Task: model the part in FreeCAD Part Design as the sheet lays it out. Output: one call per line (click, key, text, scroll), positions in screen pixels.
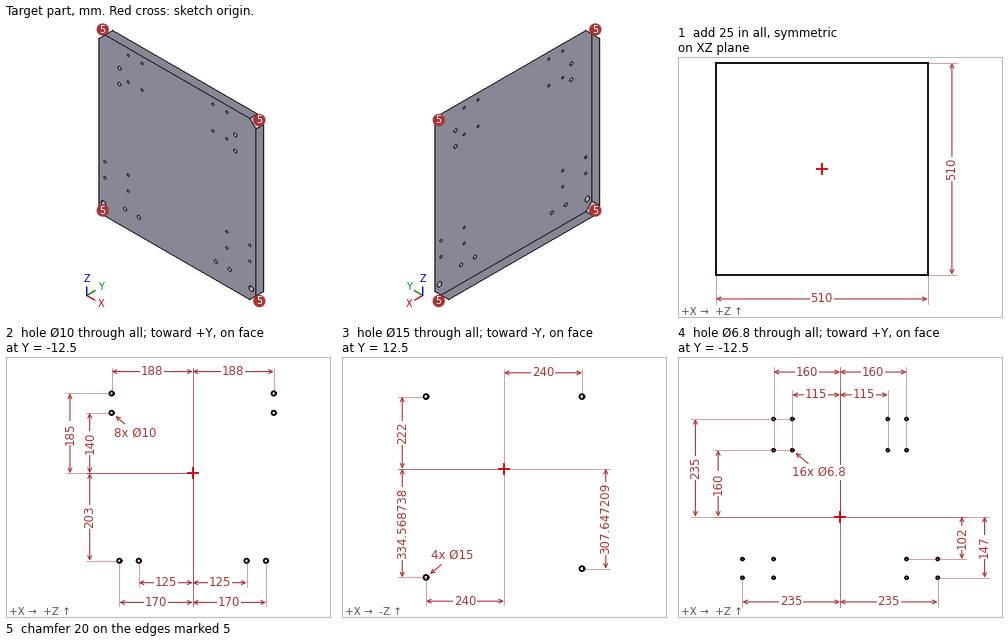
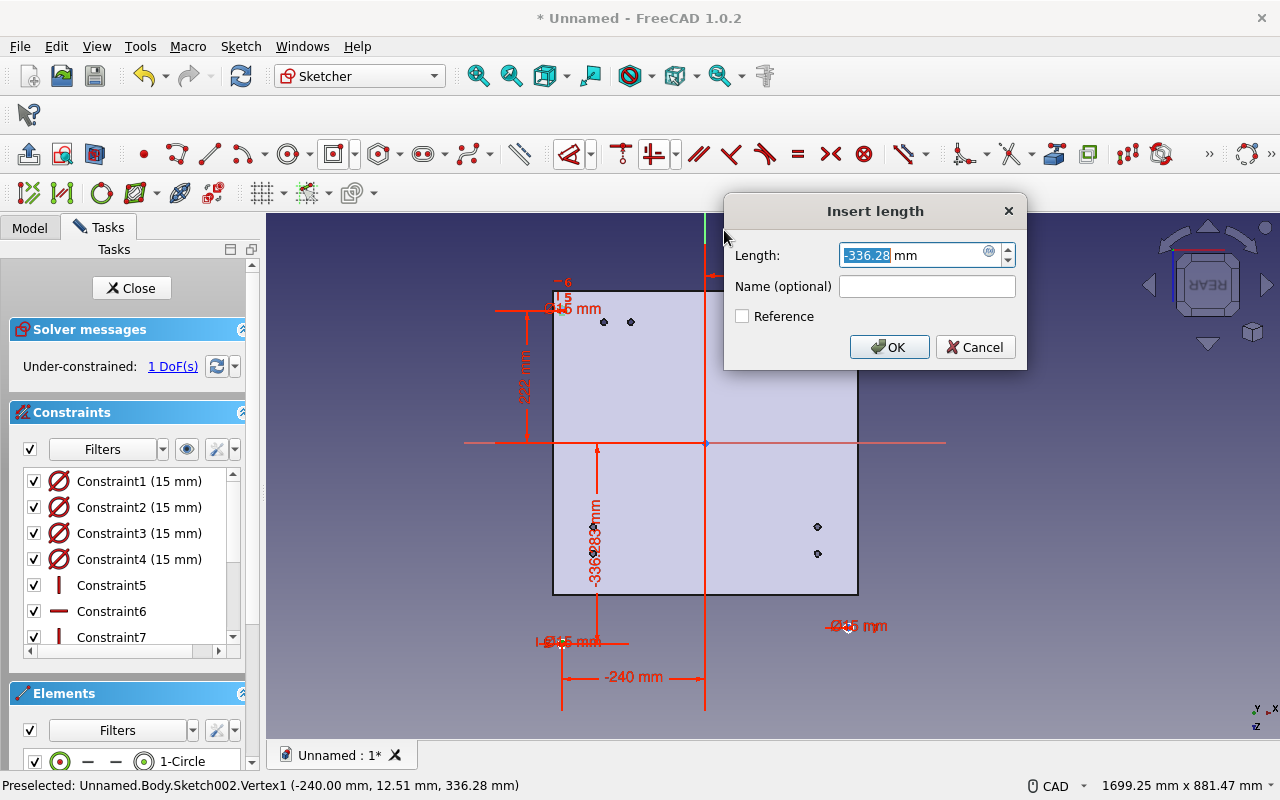
text(-334.568738)
key(Return)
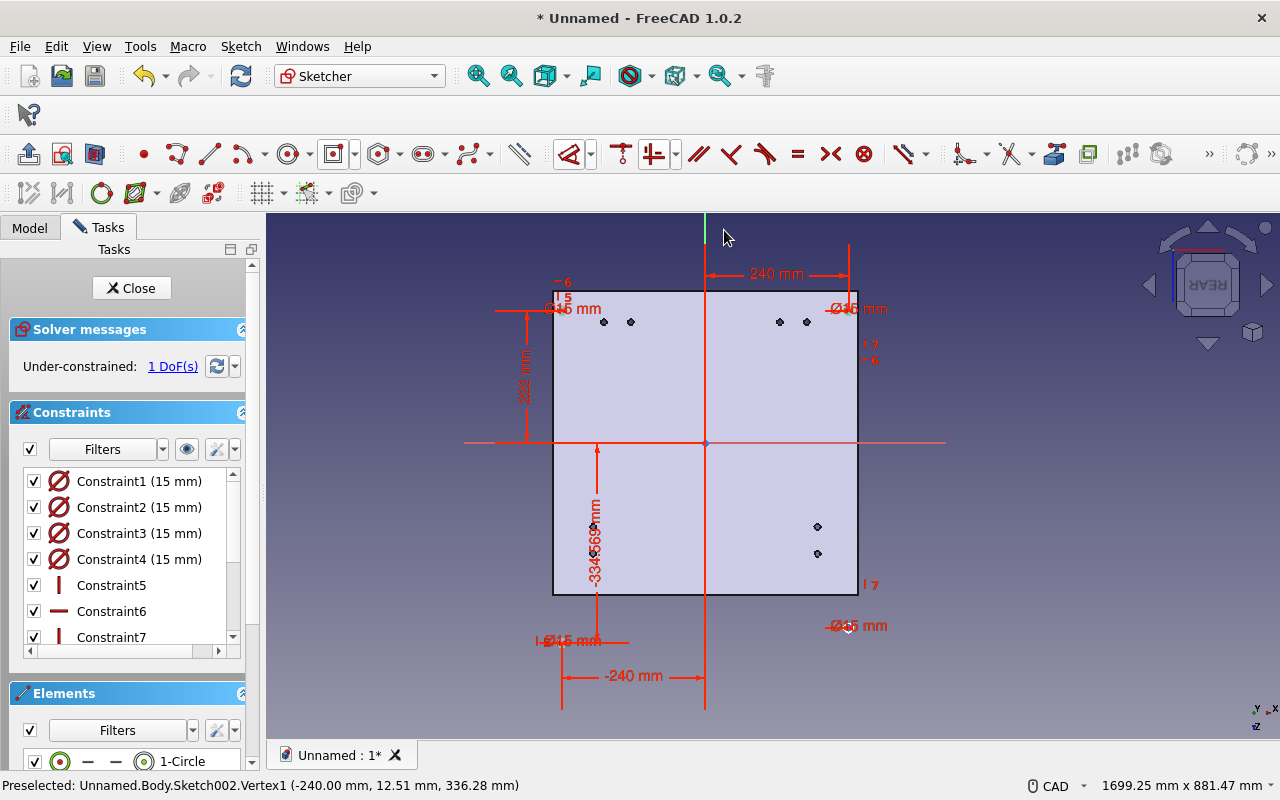
click(849, 628)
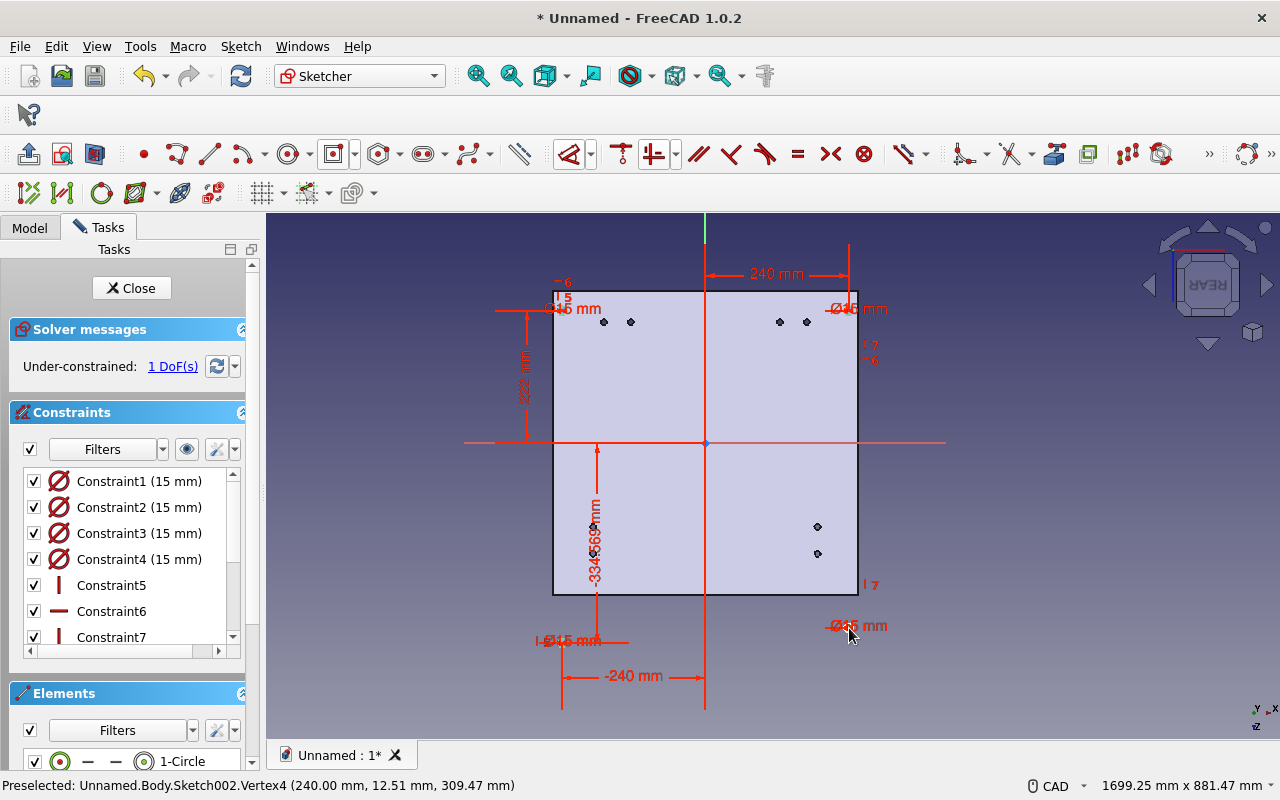
key(i)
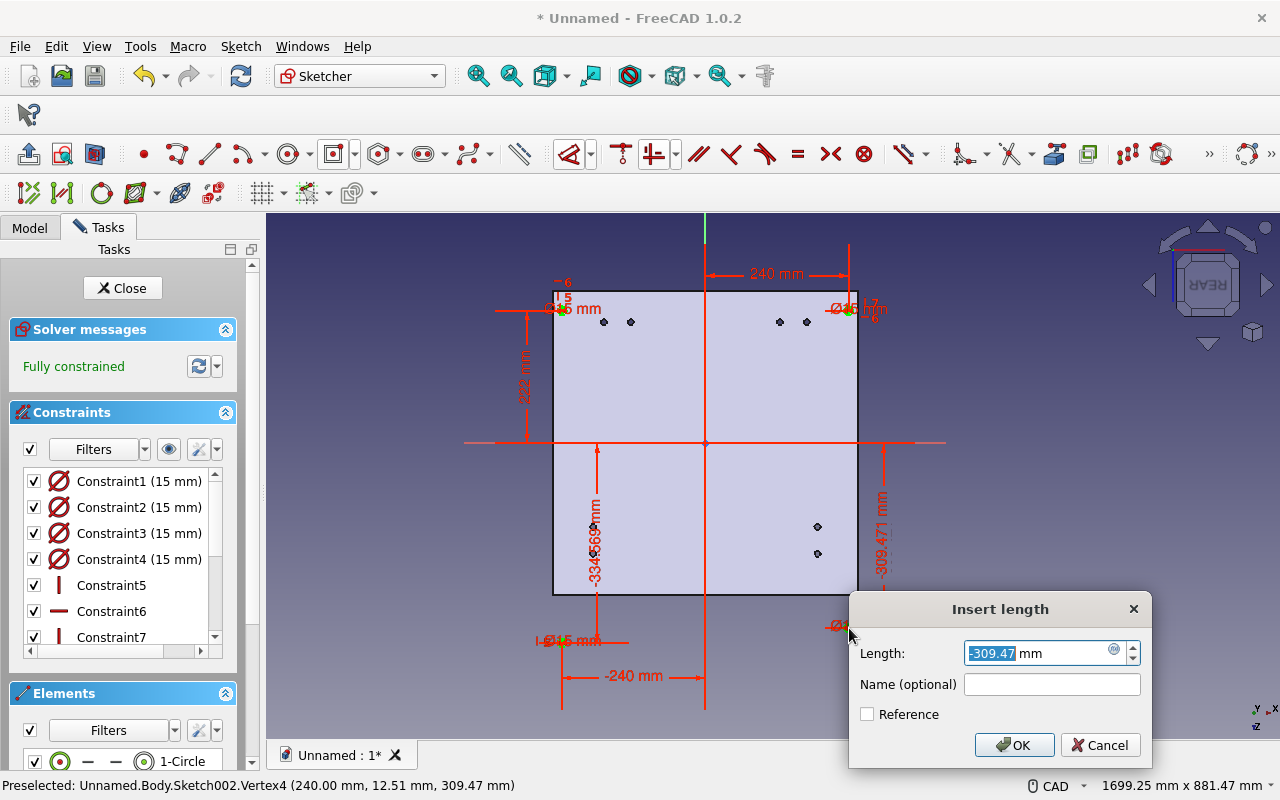
text(-307.647209)
key(Return)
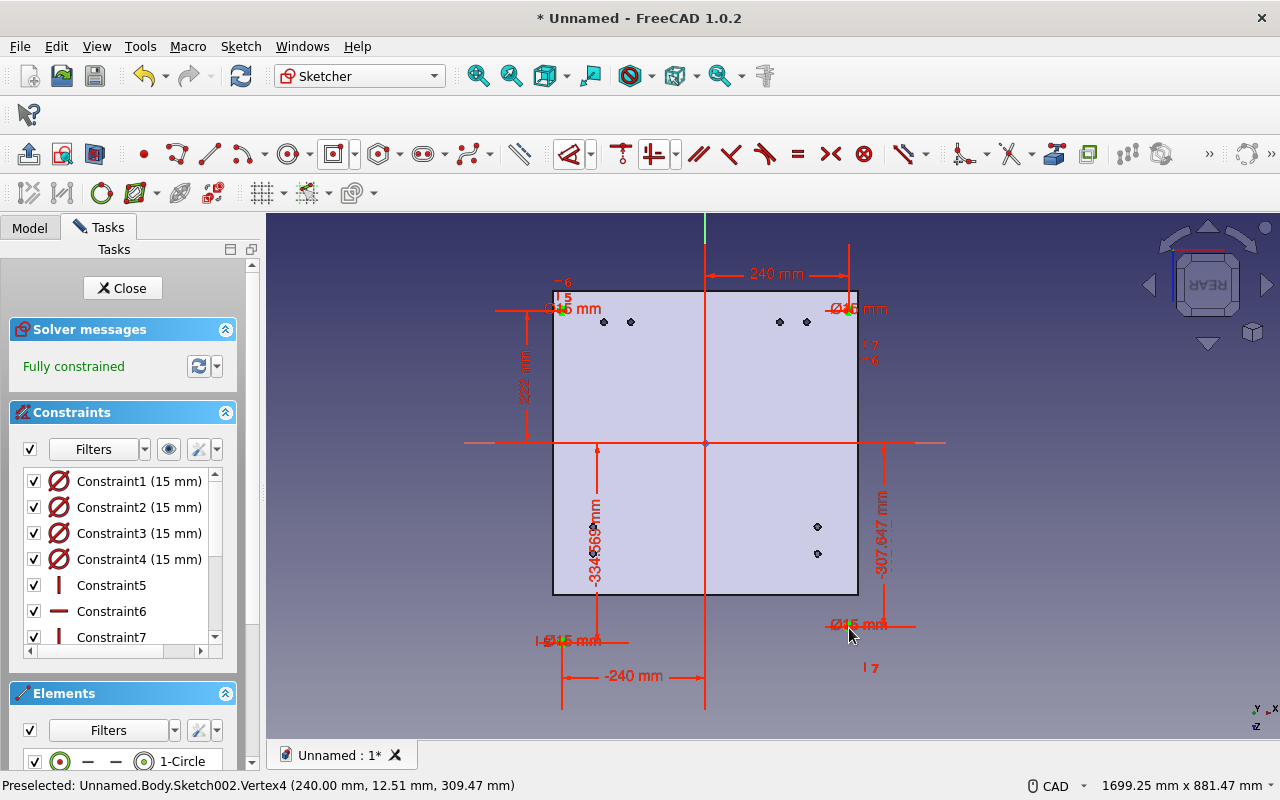
click(123, 288)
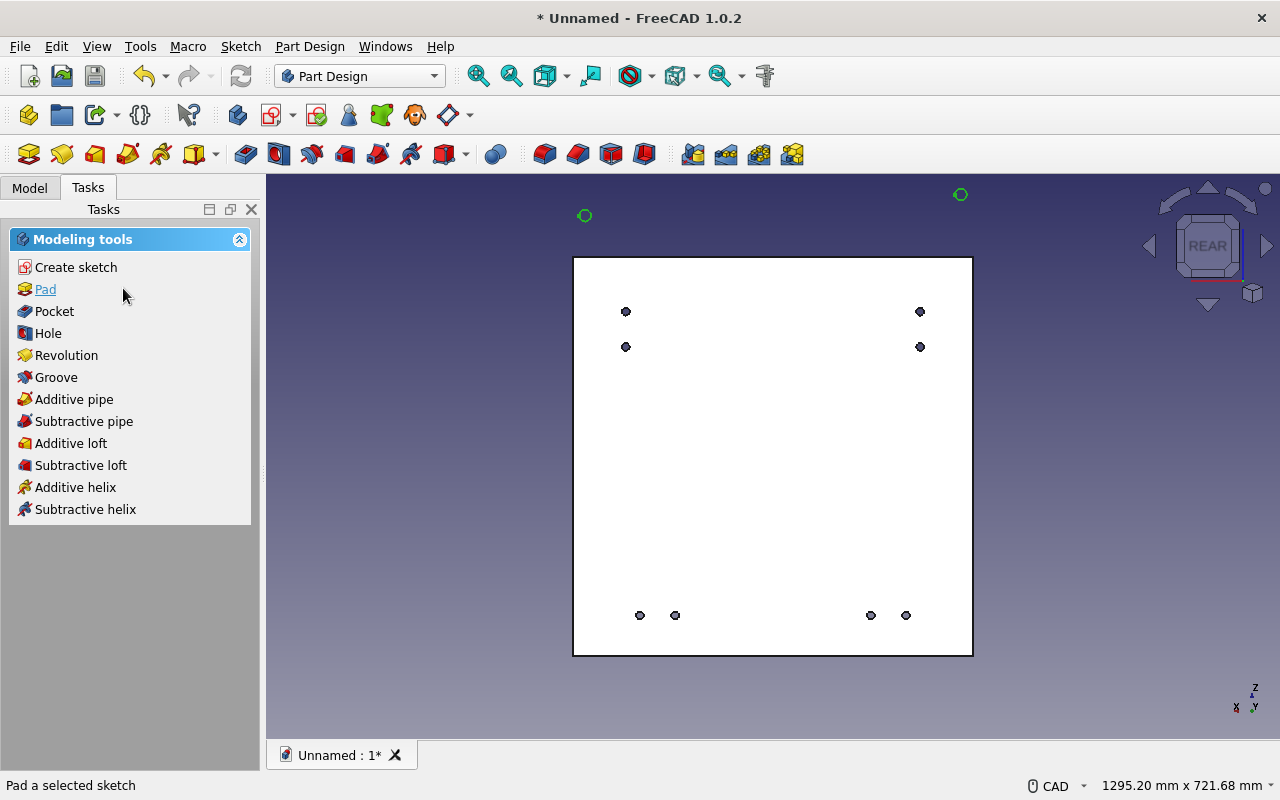
click(279, 154)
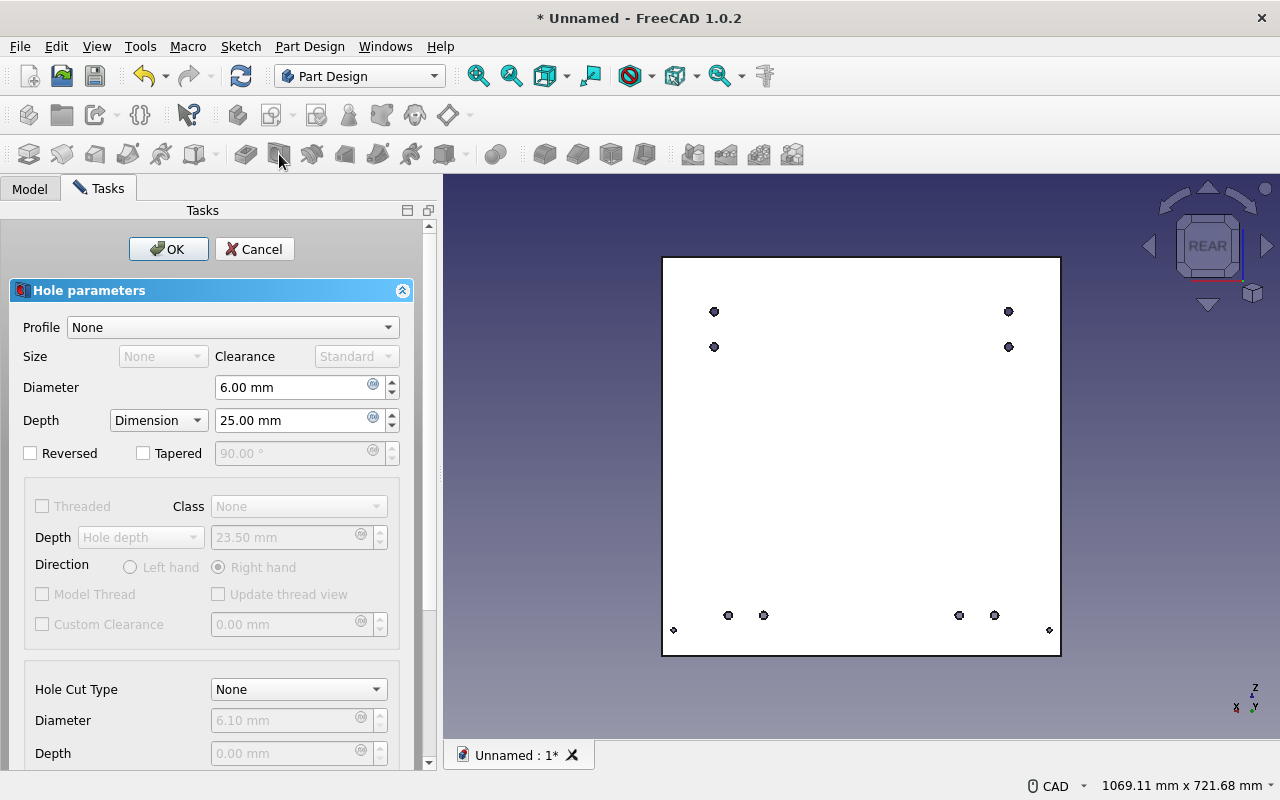
triple_click(300, 388)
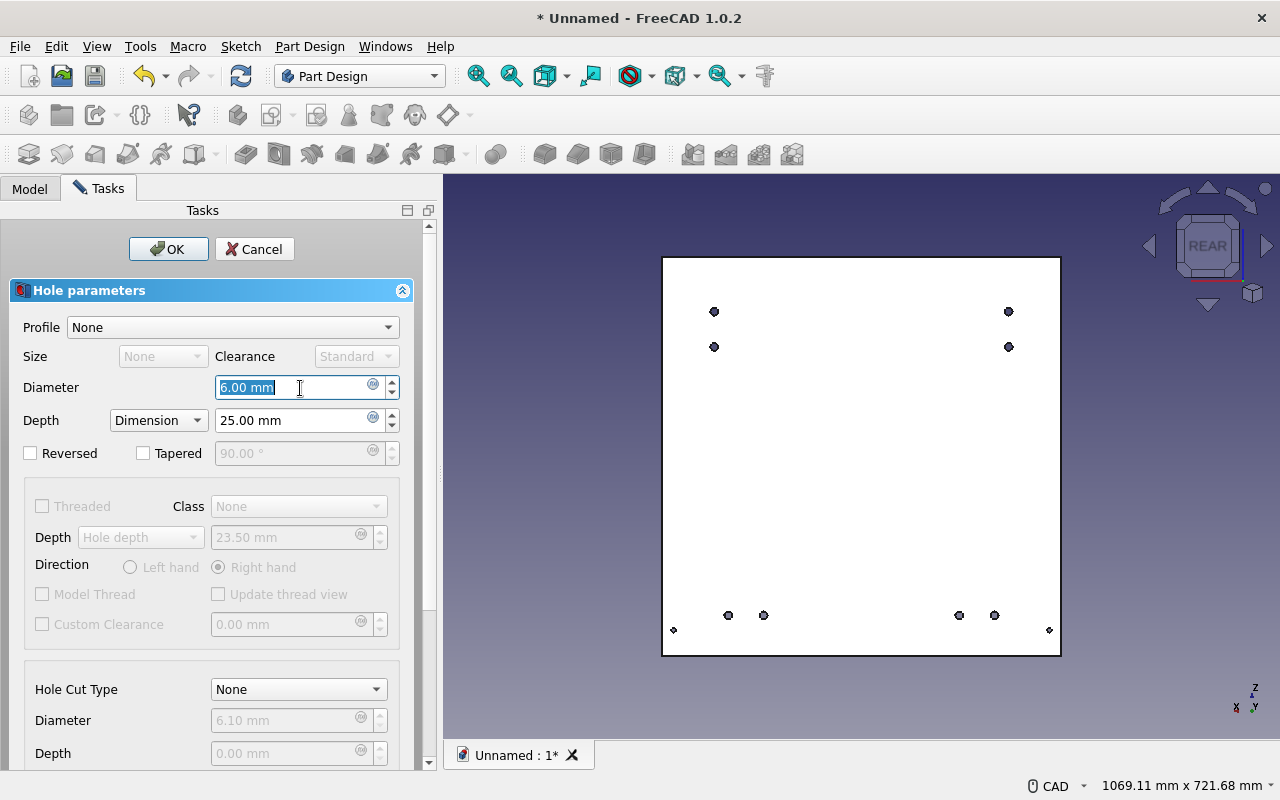
text(15)
key(Tab)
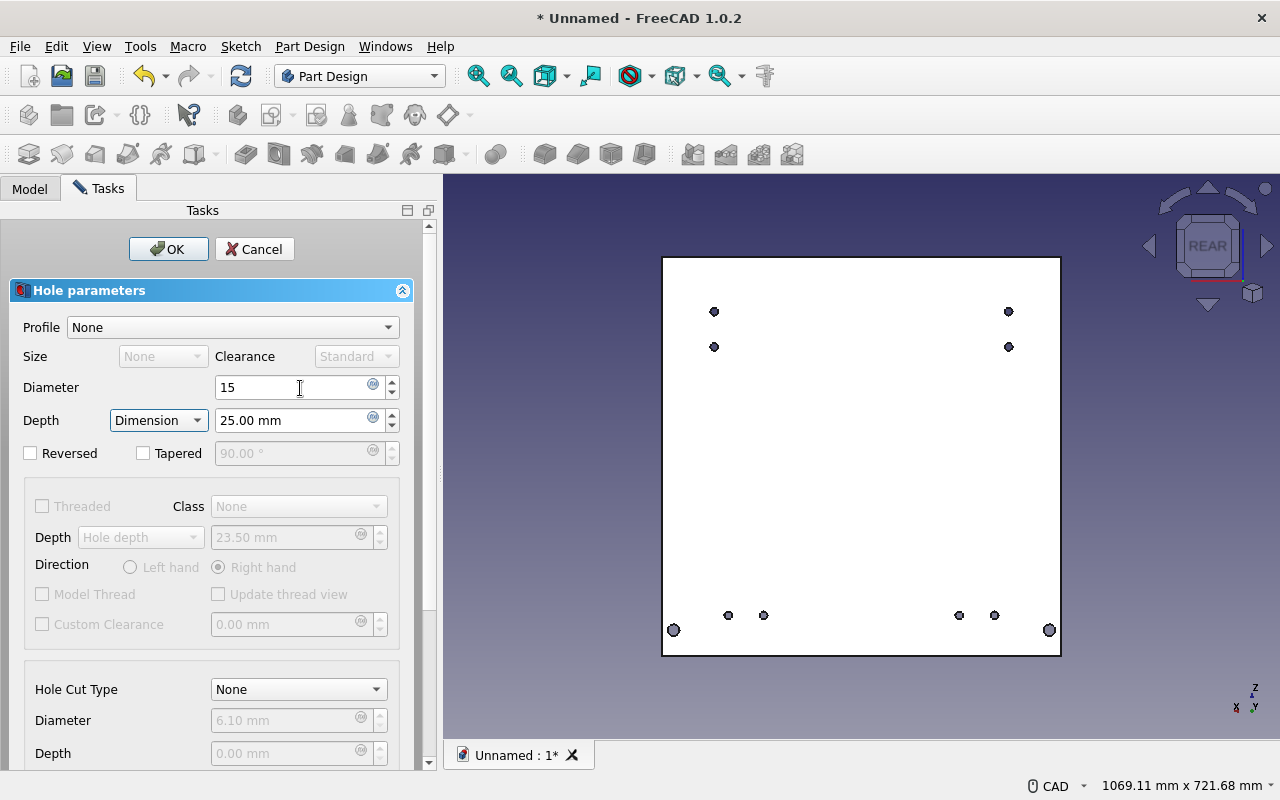
click(160, 420)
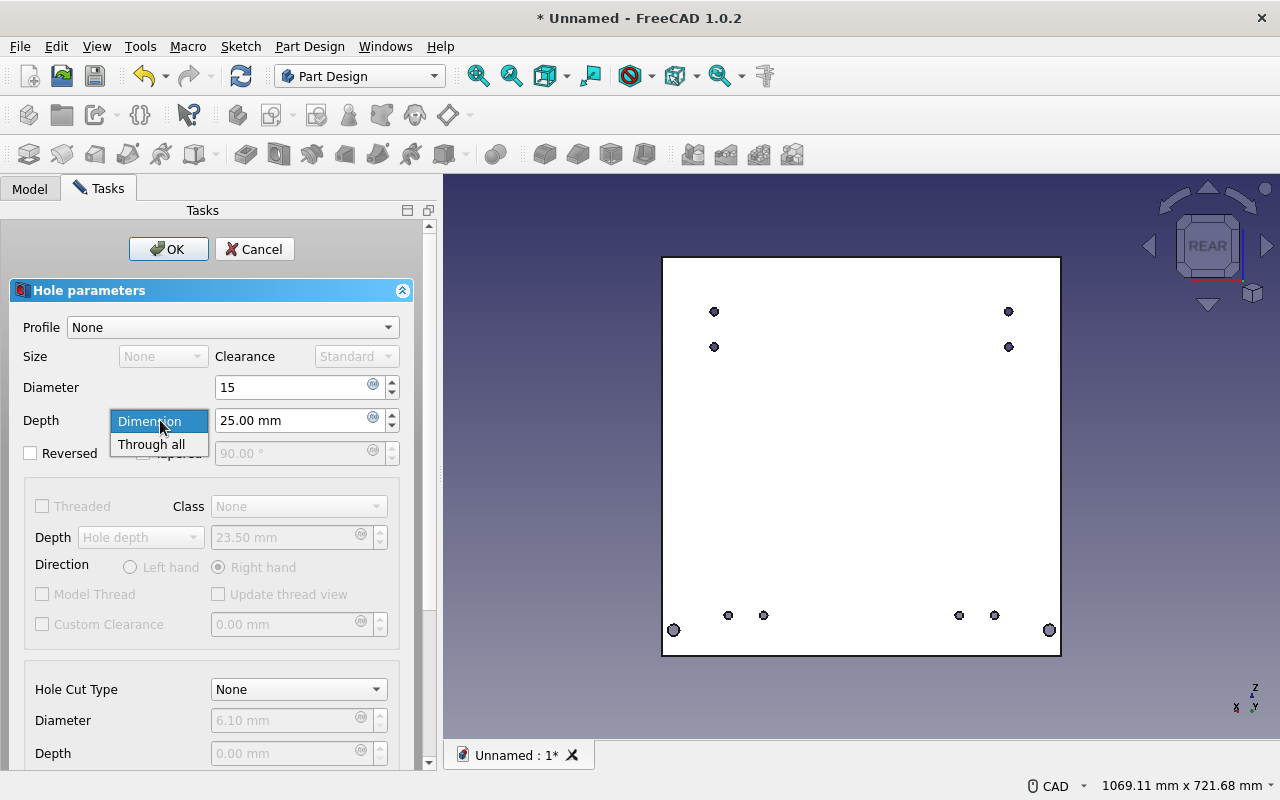
click(158, 444)